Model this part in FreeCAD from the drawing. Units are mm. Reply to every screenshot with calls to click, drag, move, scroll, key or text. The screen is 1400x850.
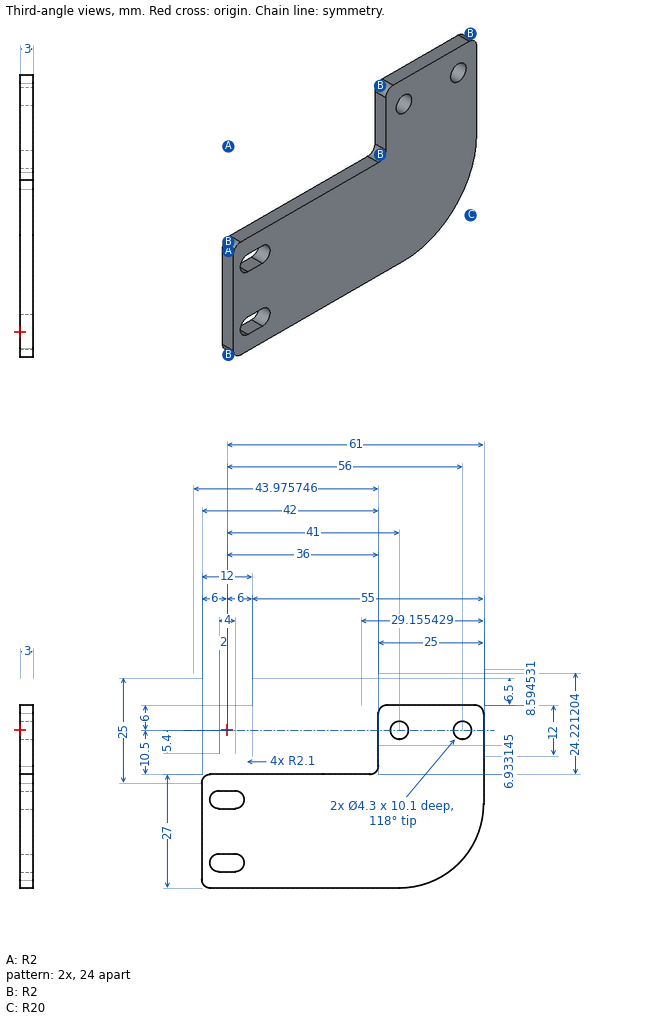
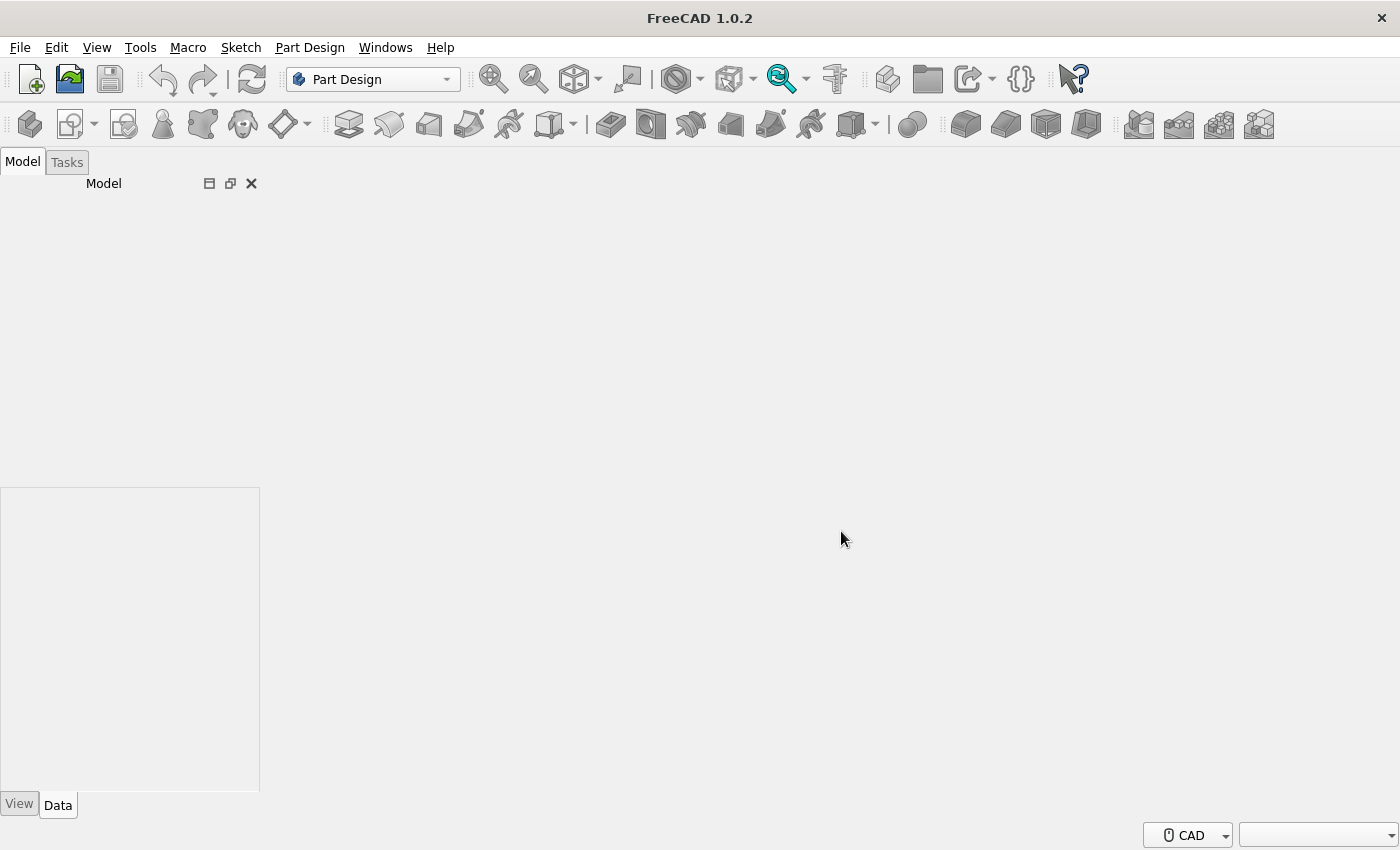
key(ctrl+n)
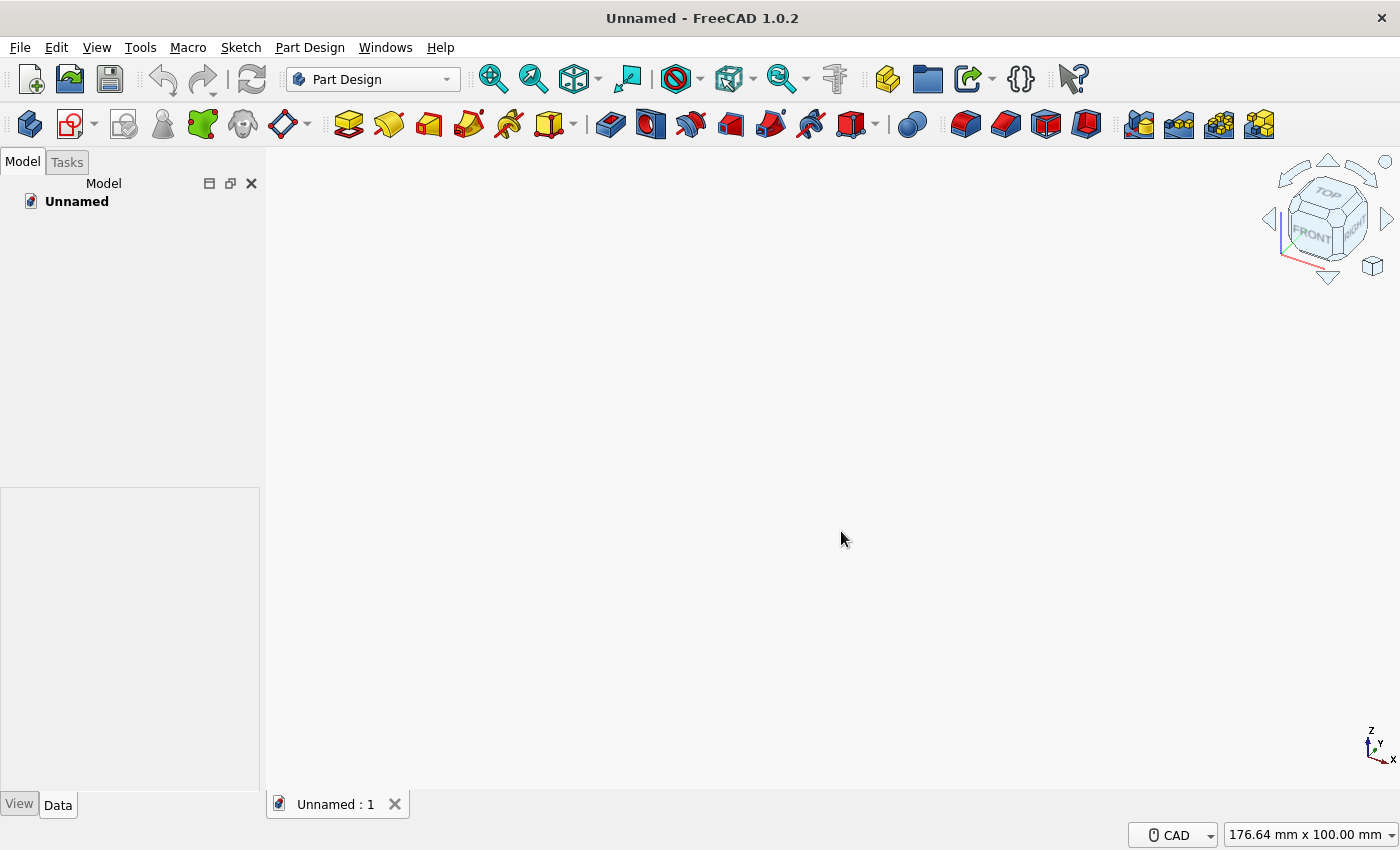
click(70, 124)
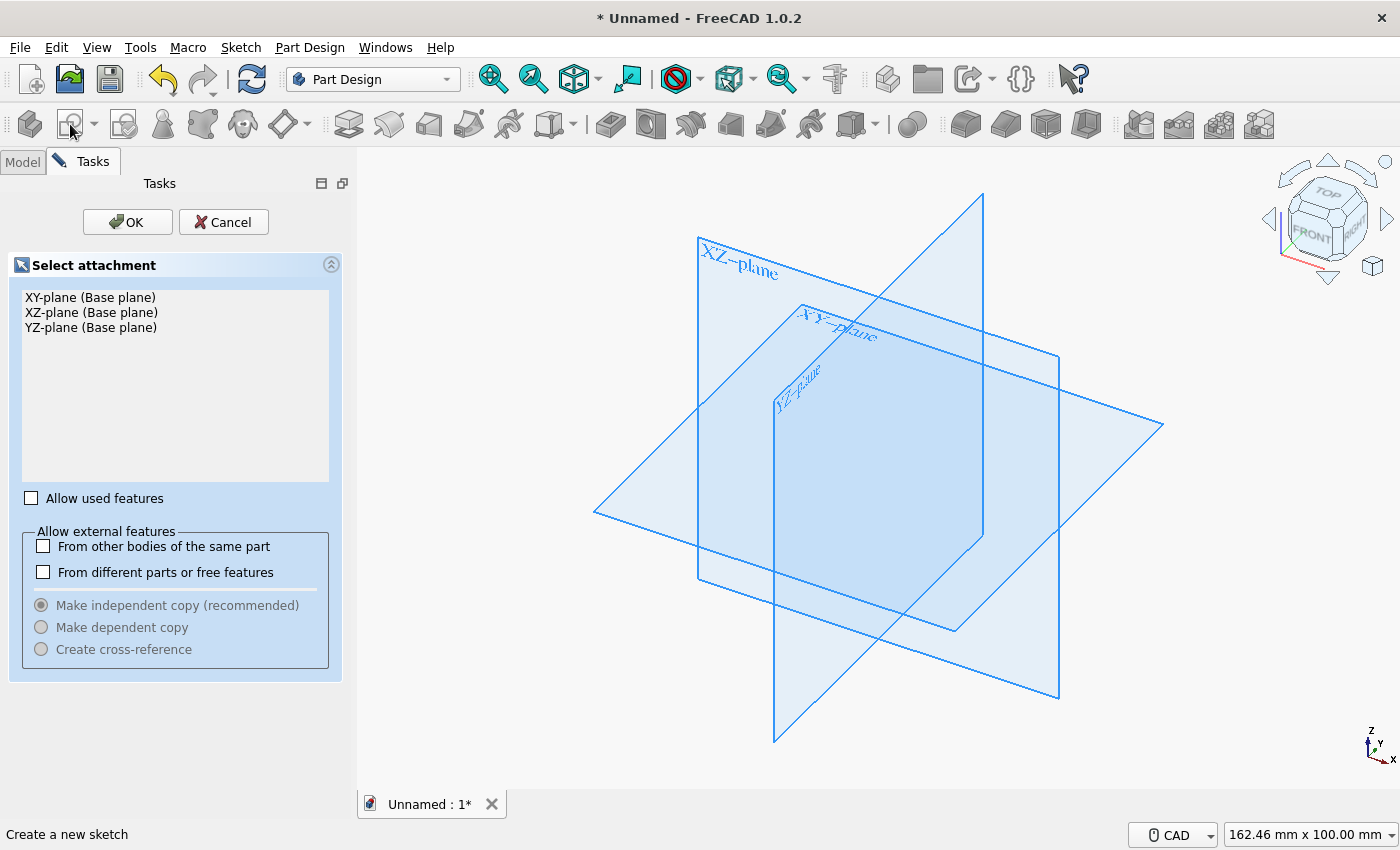
click(82, 328)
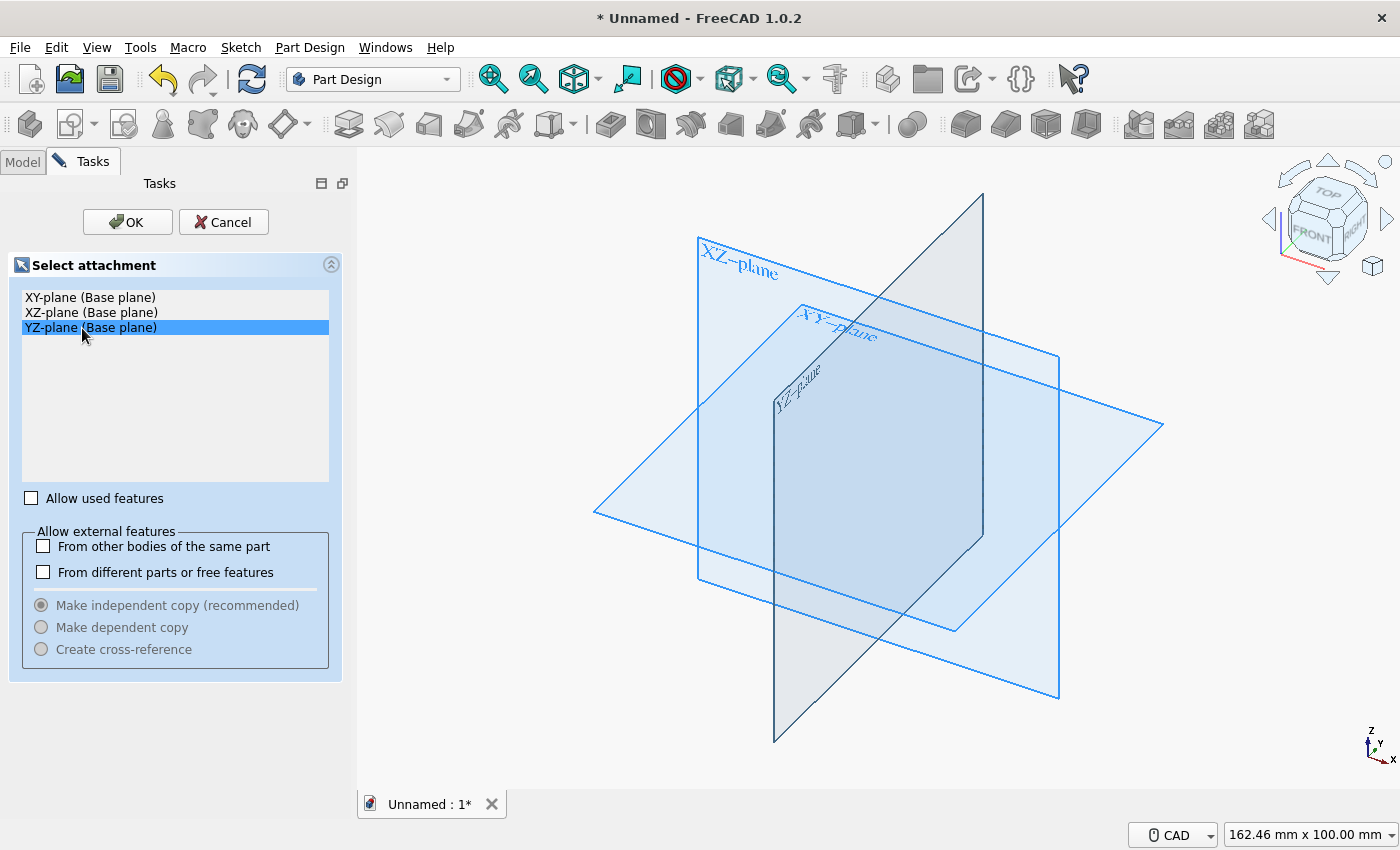
click(128, 222)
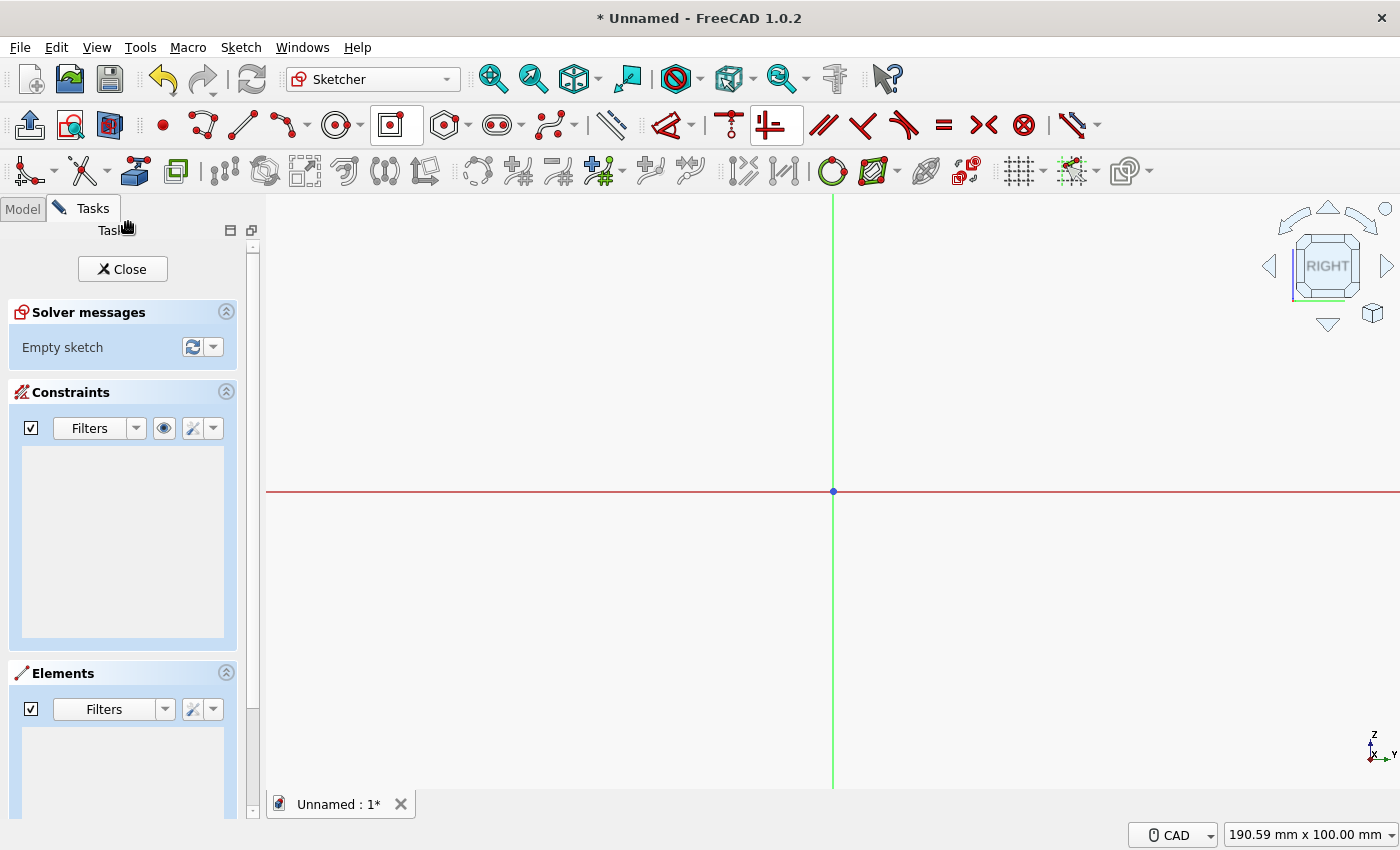
scroll(1235, 492, up, 3)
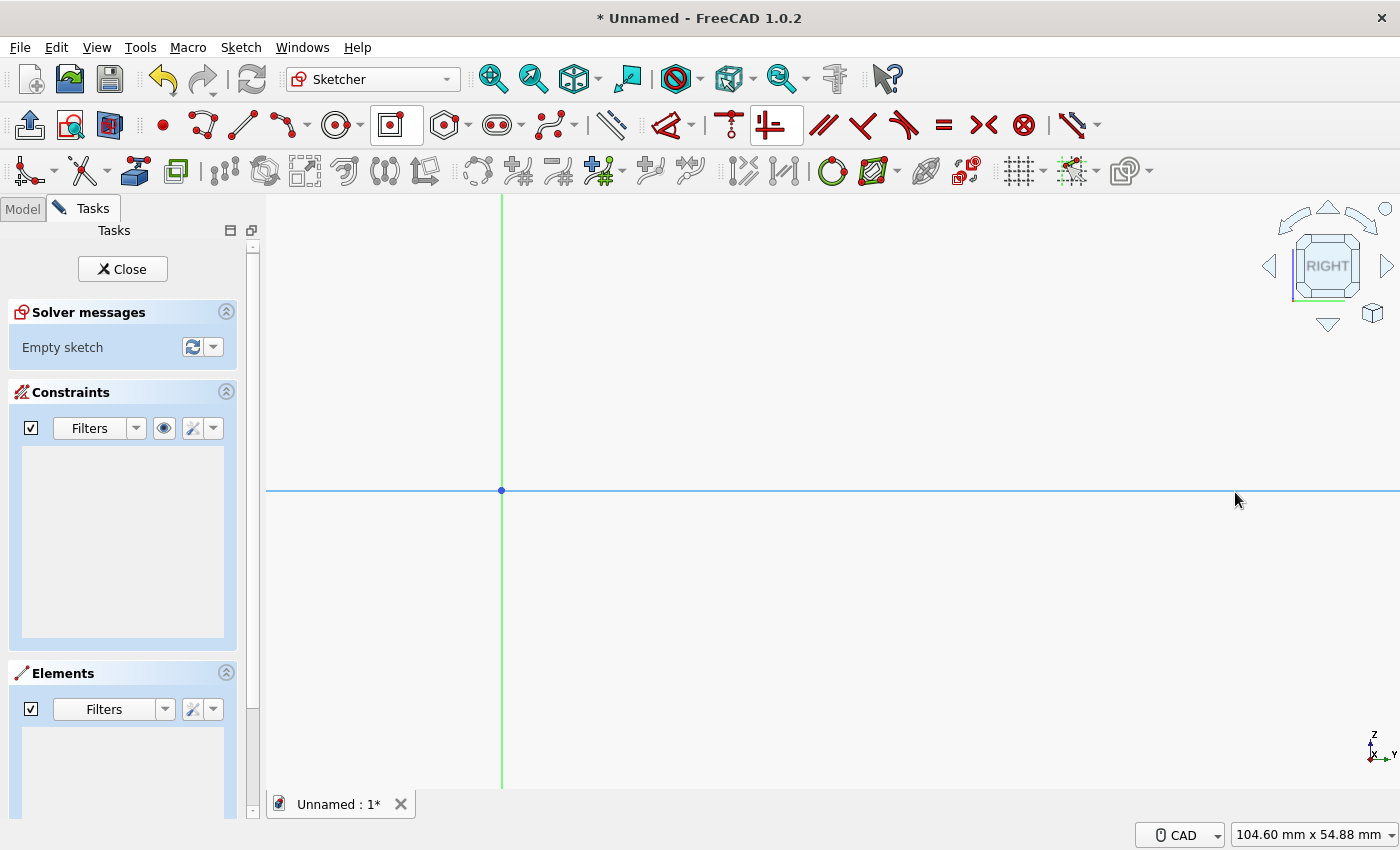
click(204, 126)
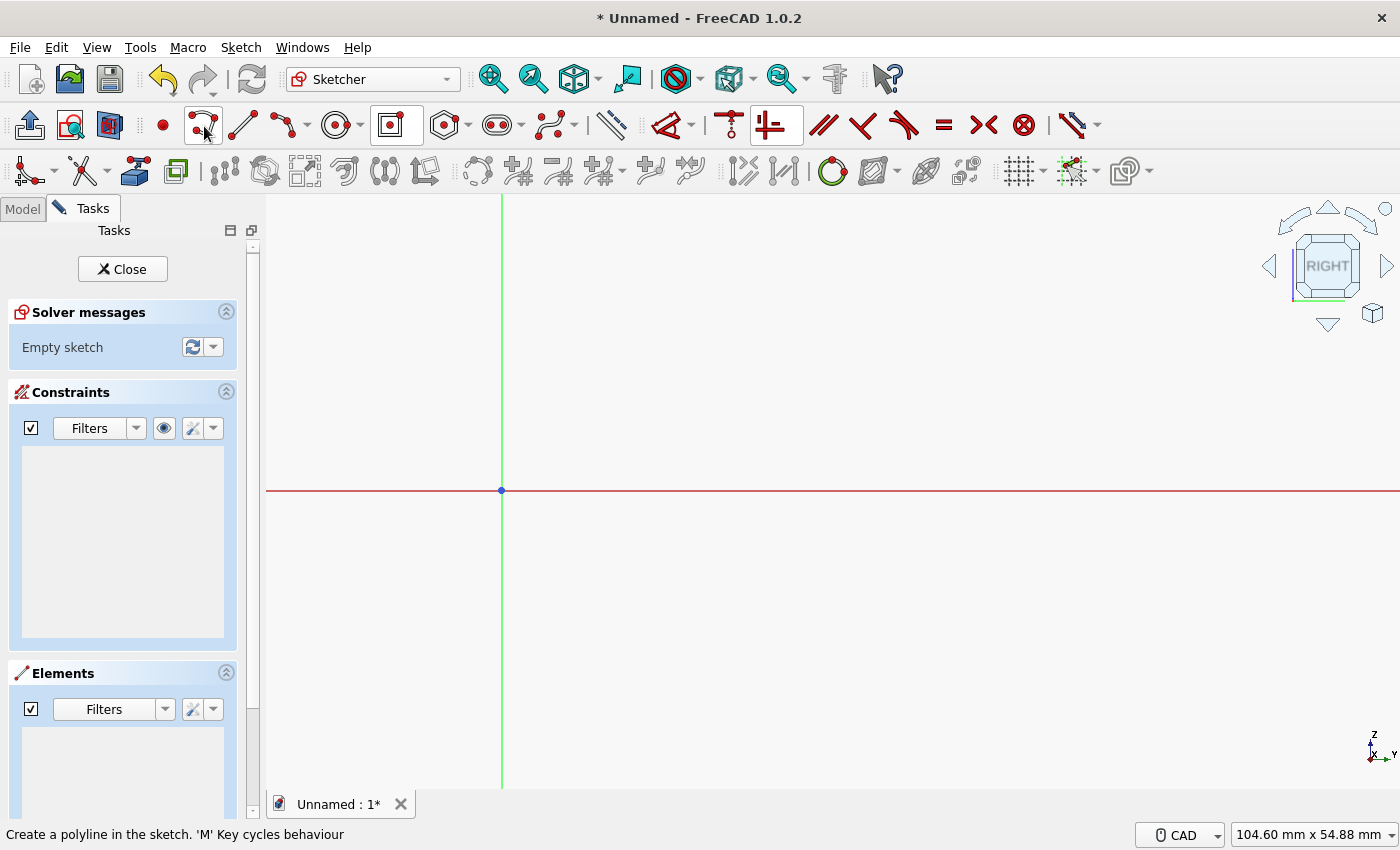
click(567, 426)
click(567, 355)
click(437, 355)
click(437, 626)
click(567, 626)
click(567, 556)
click(1163, 556)
click(1163, 426)
click(567, 427)
key(Escape)
key(Escape)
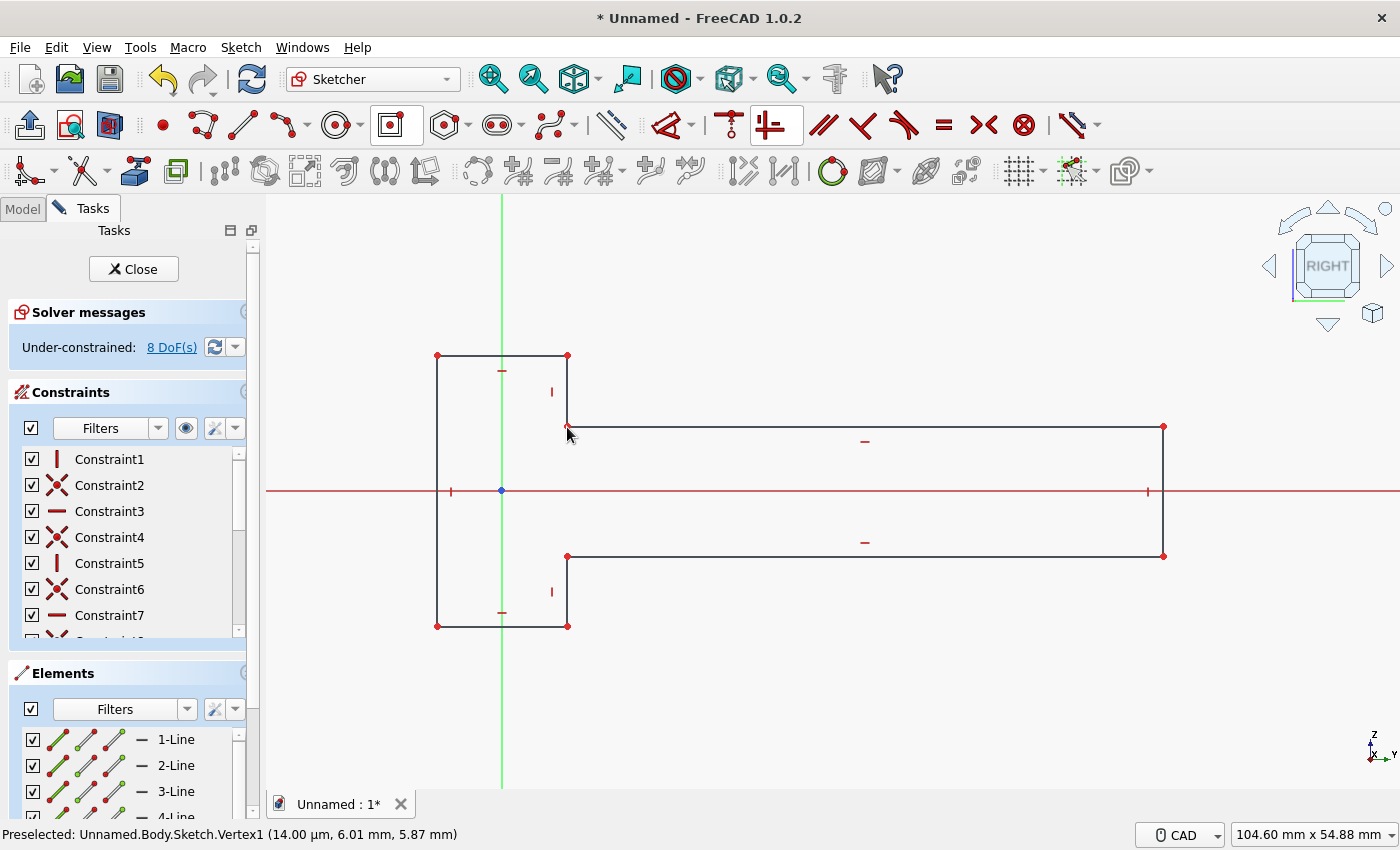
click(567, 356)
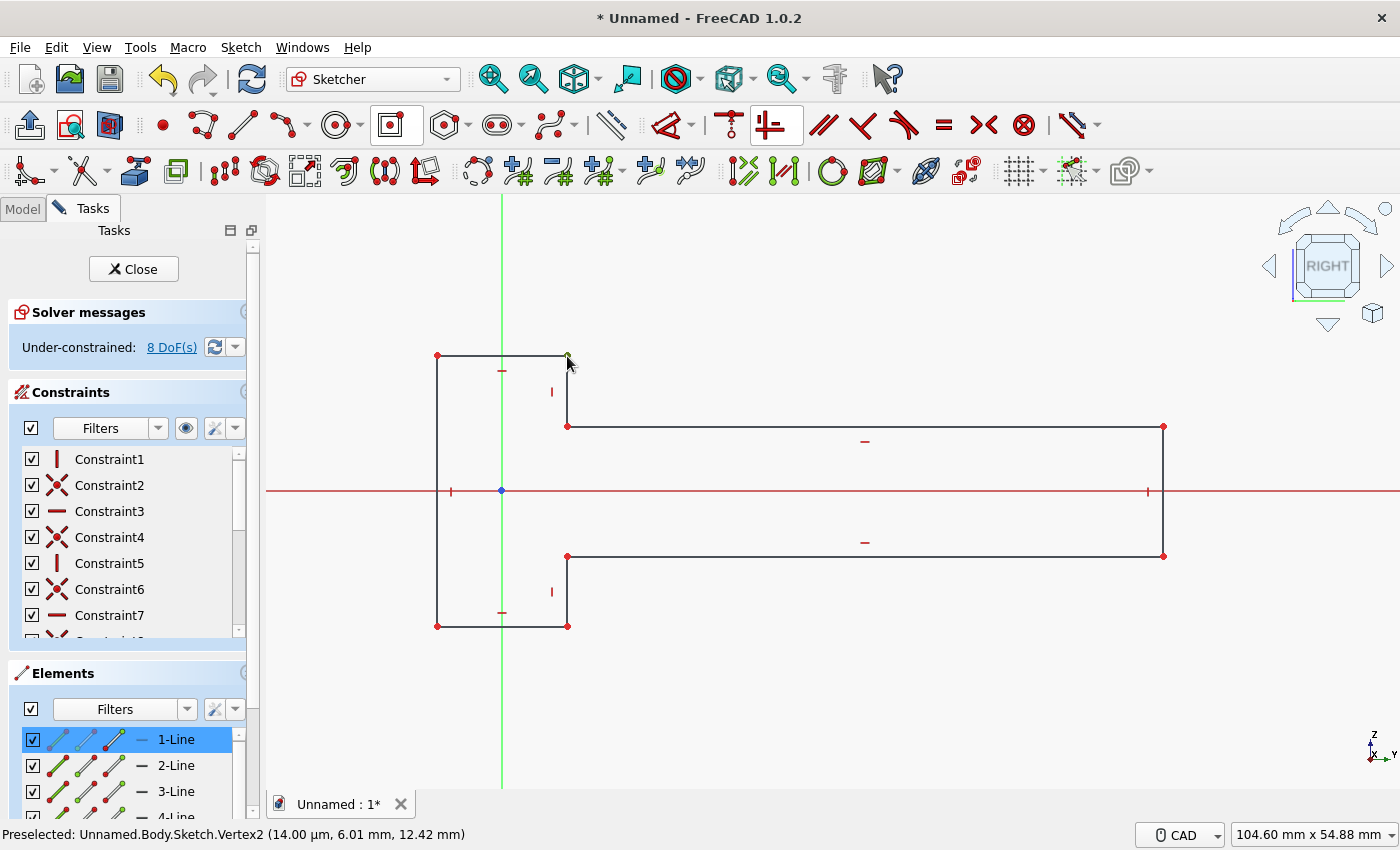
click(567, 627)